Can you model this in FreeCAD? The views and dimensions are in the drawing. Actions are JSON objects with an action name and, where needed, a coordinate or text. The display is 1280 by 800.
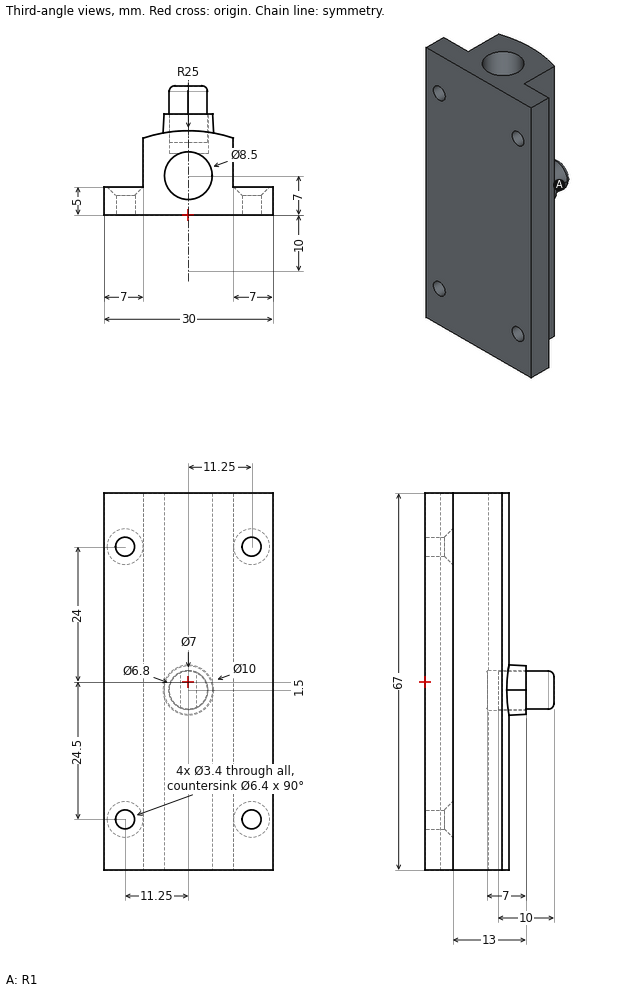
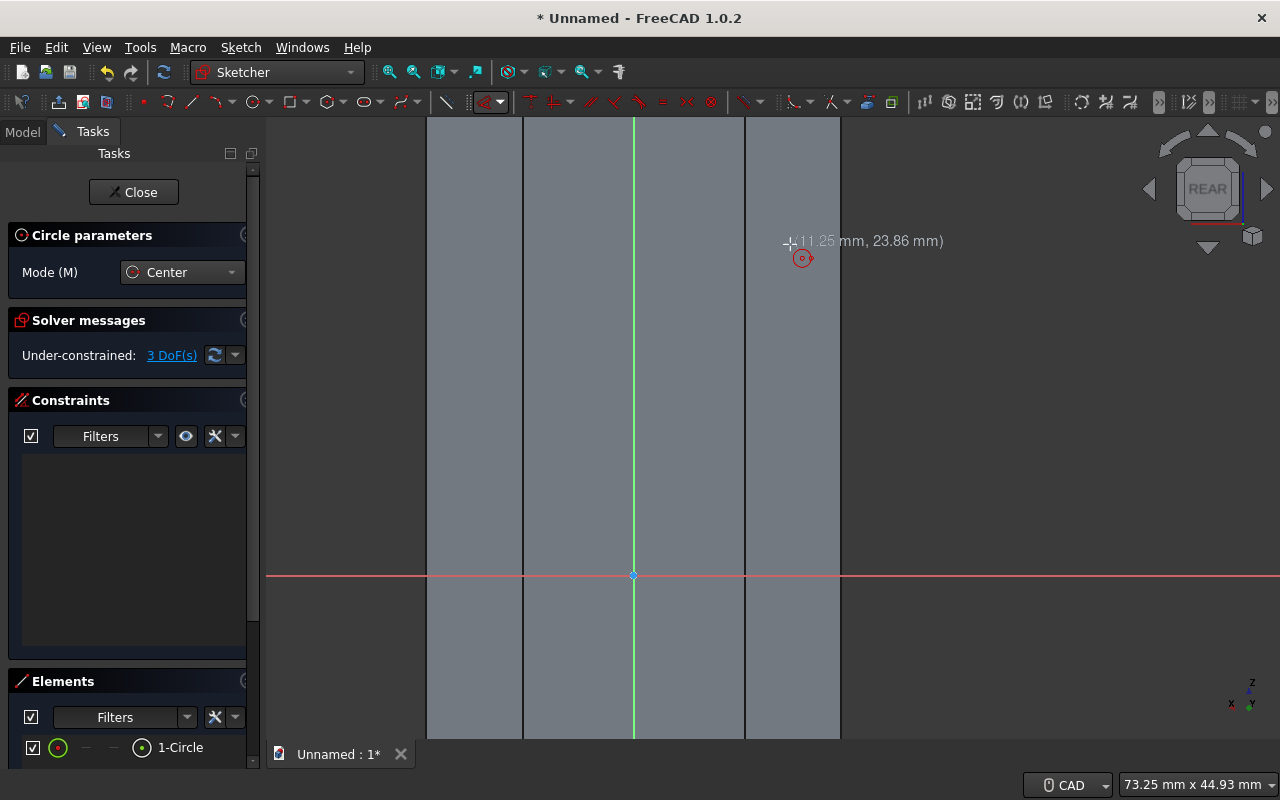
{"action": "left_click", "coordinate": [790, 244]}
{"action": "left_click", "coordinate": [806, 227]}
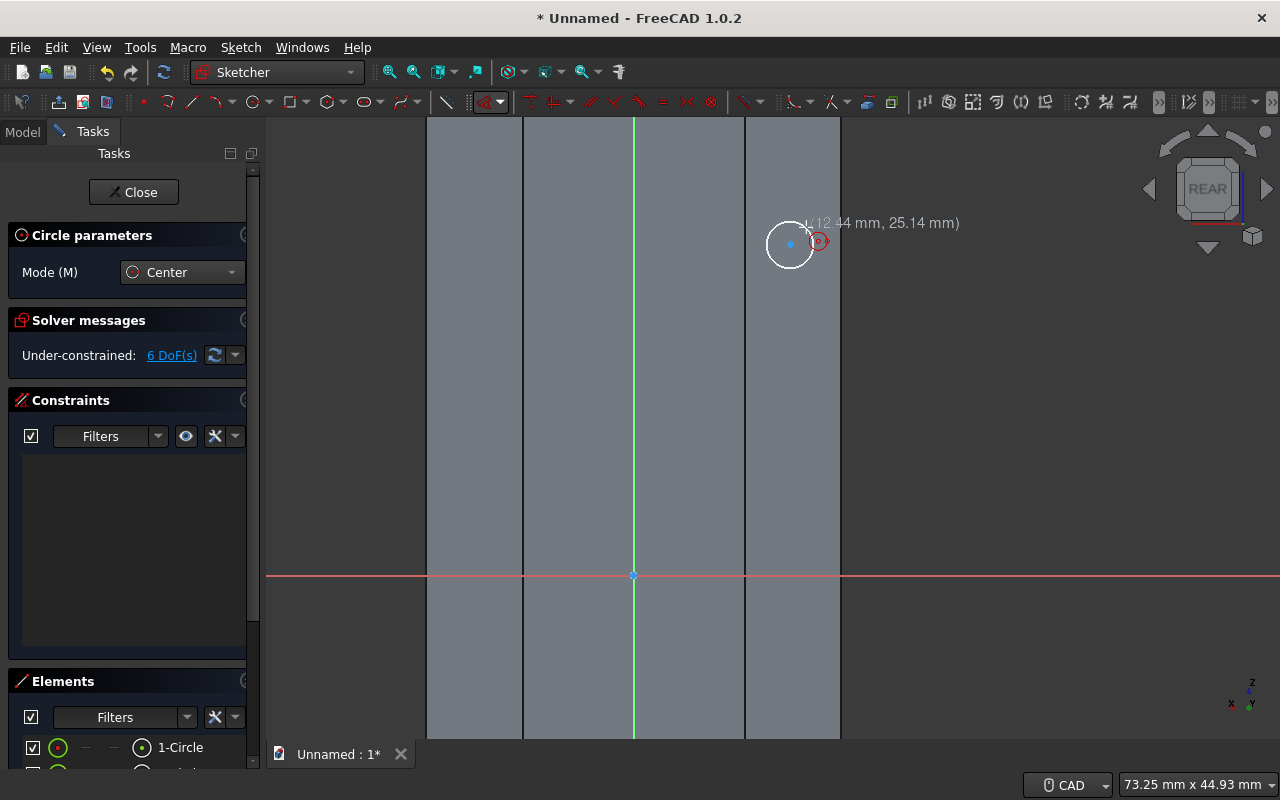
{"action": "left_click", "coordinate": [478, 244]}
{"action": "left_click", "coordinate": [495, 227]}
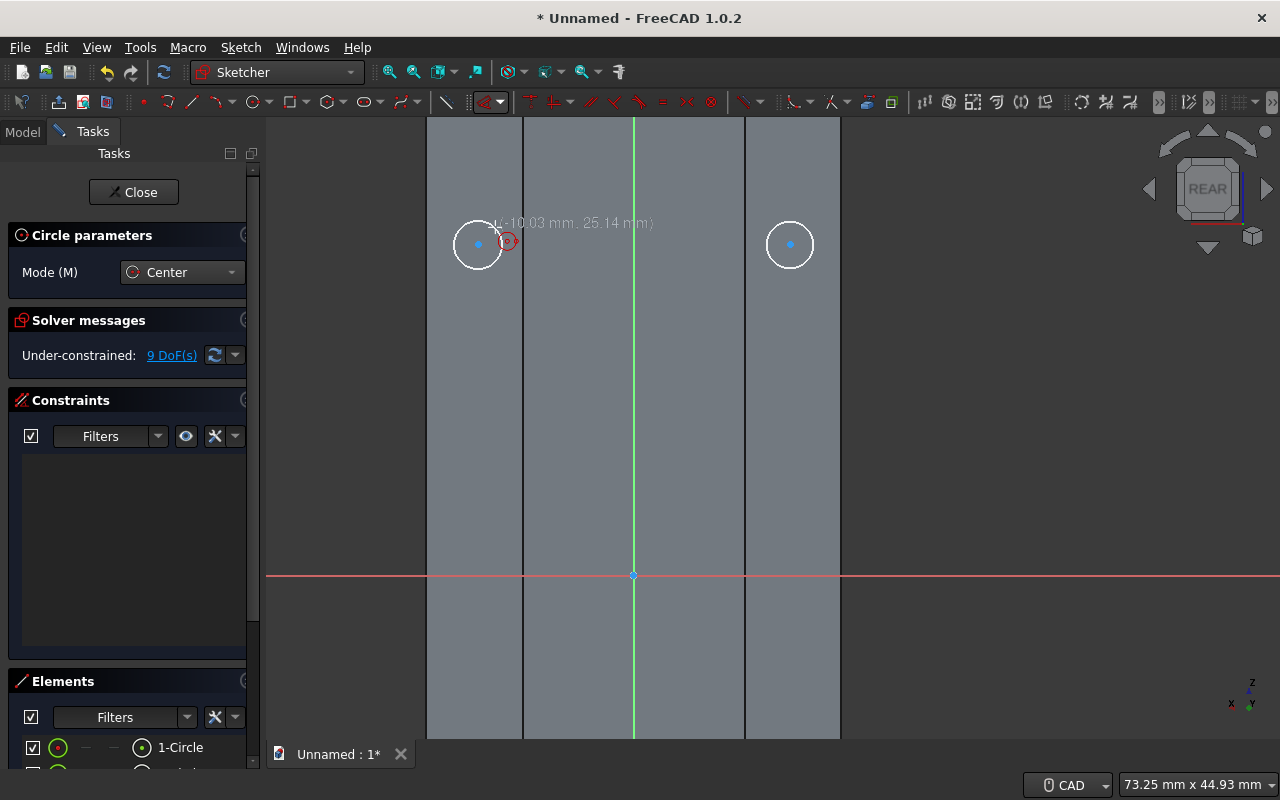
{"action": "scroll", "coordinate": [790, 244], "scroll_direction": "down", "scroll_amount": 3}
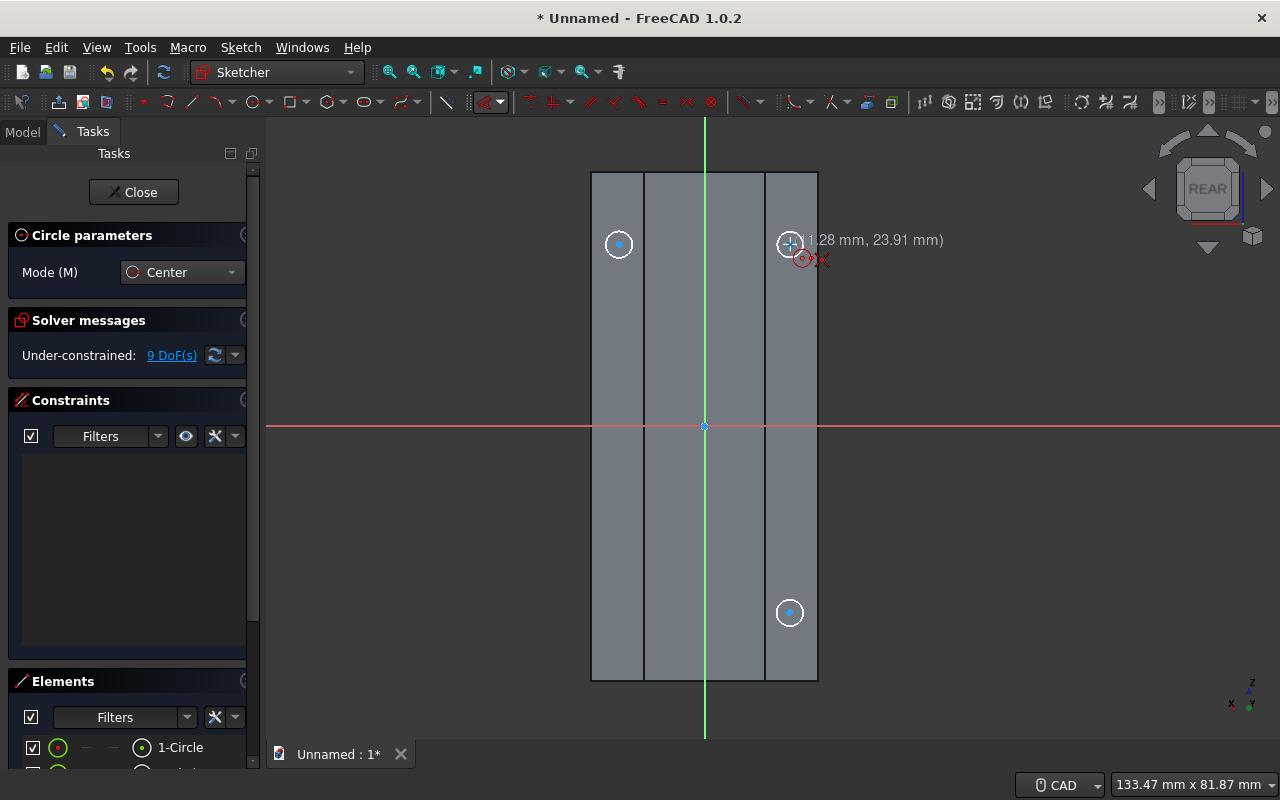
{"action": "scroll", "coordinate": [619, 612], "scroll_direction": "up", "scroll_amount": 3}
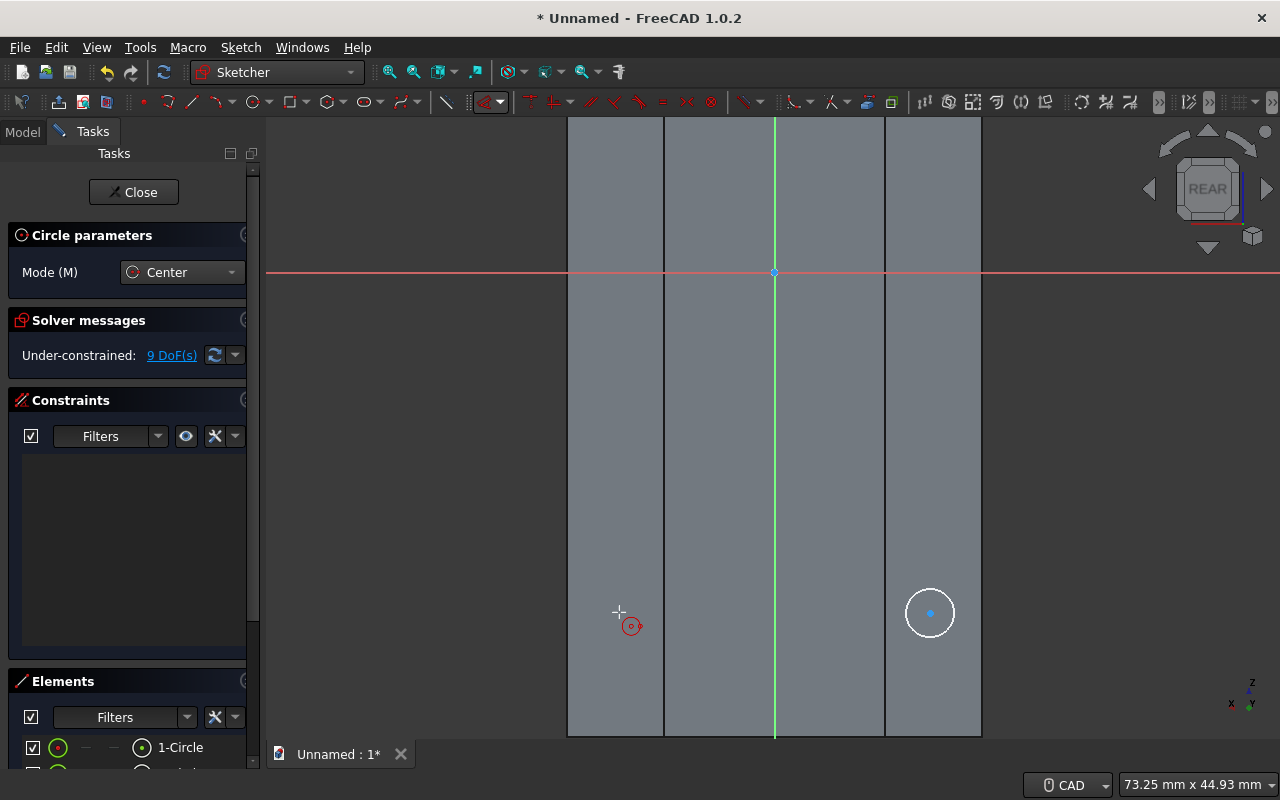
{"action": "left_click", "coordinate": [619, 612]}
{"action": "left_click", "coordinate": [635, 595]}
{"action": "key", "text": "Escape"}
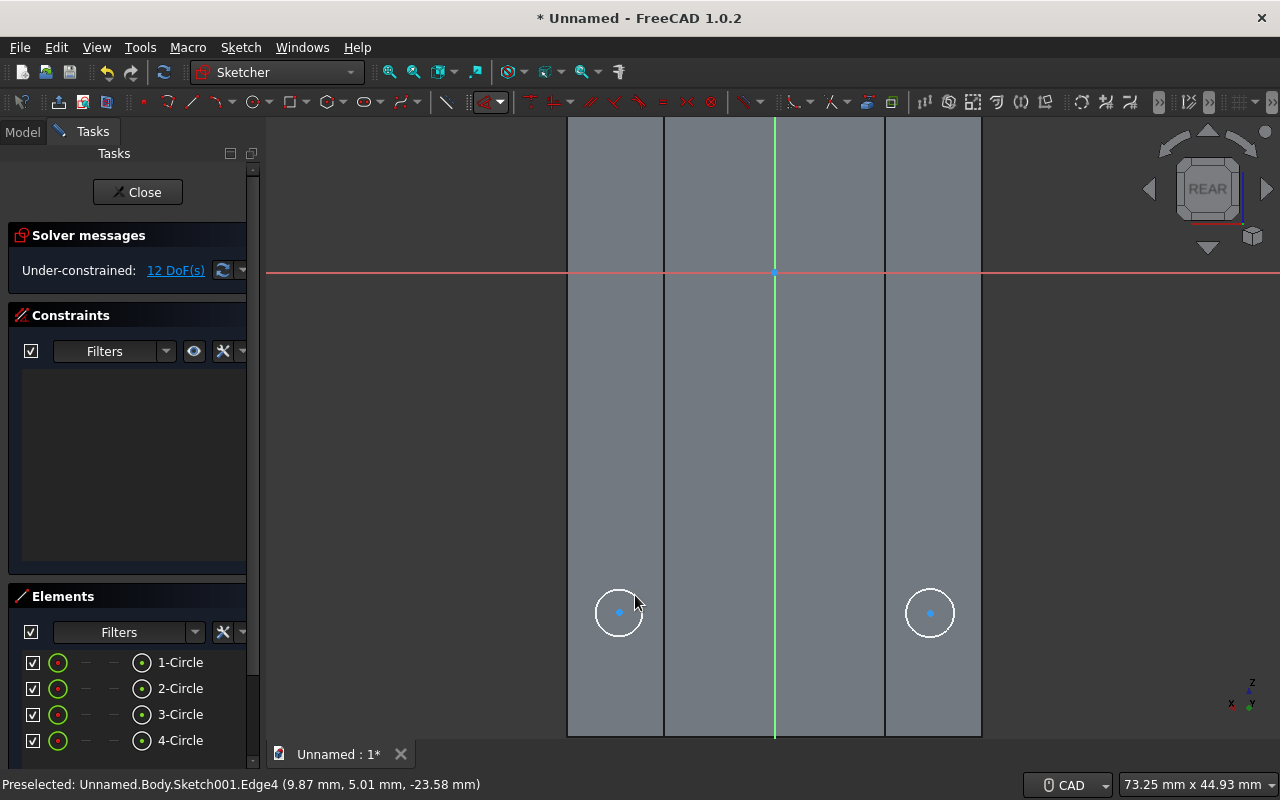
{"action": "left_click", "coordinate": [947, 596]}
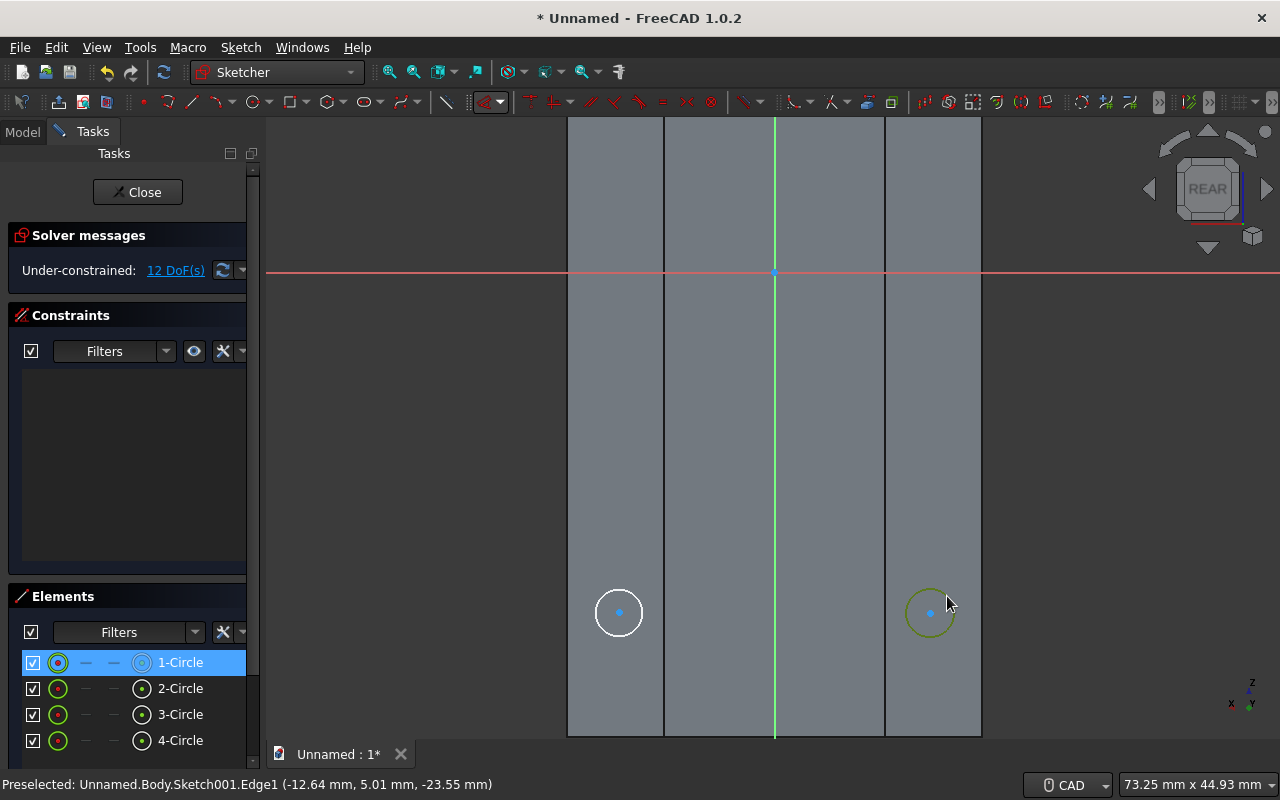
{"action": "scroll", "coordinate": [619, 612], "scroll_direction": "down", "scroll_amount": 3}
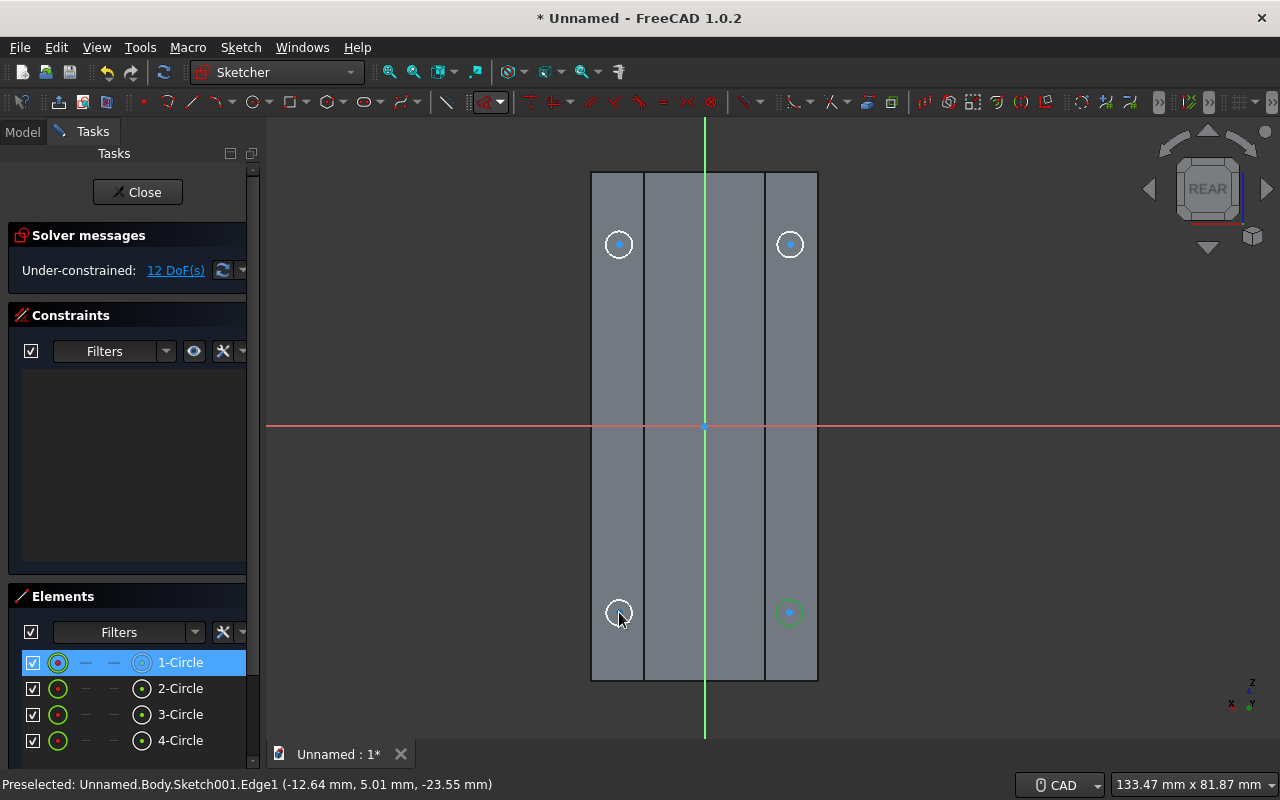
{"action": "left_click", "coordinate": [799, 236]}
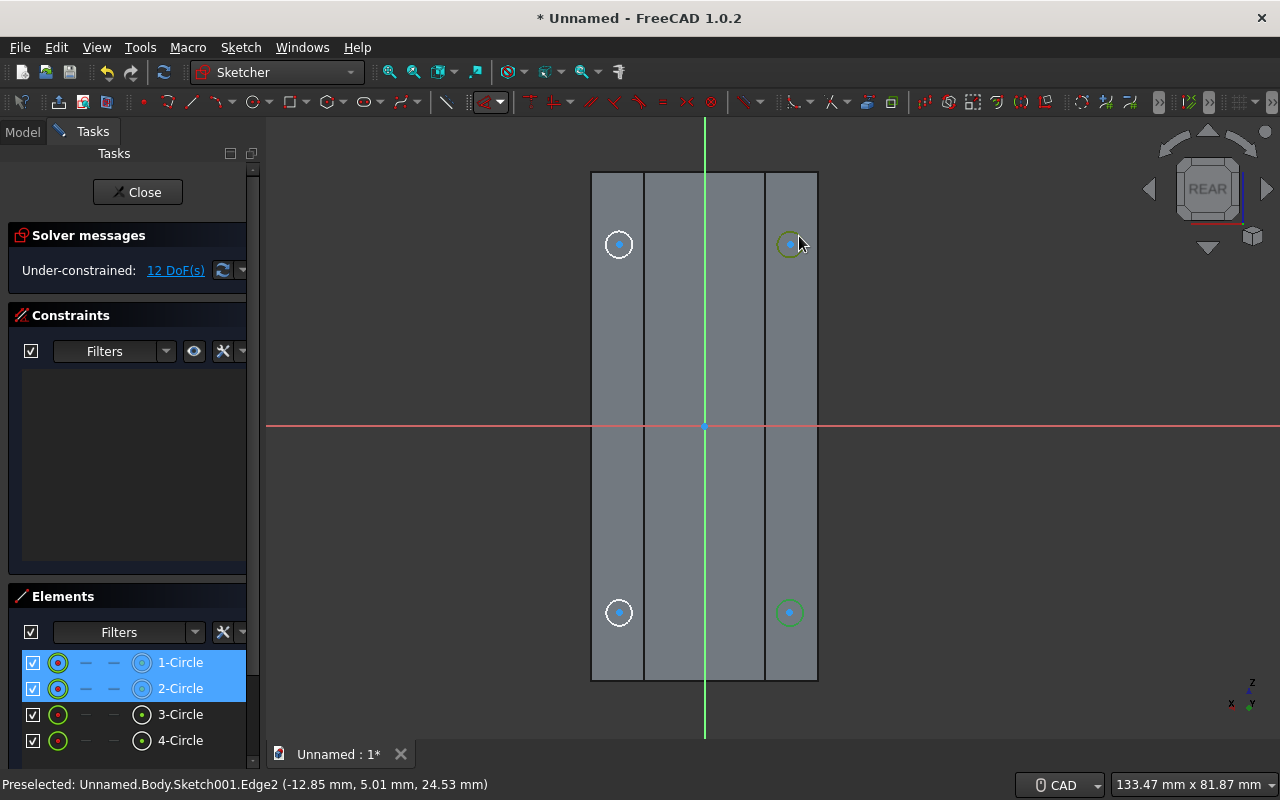
{"action": "left_click", "coordinate": [628, 235]}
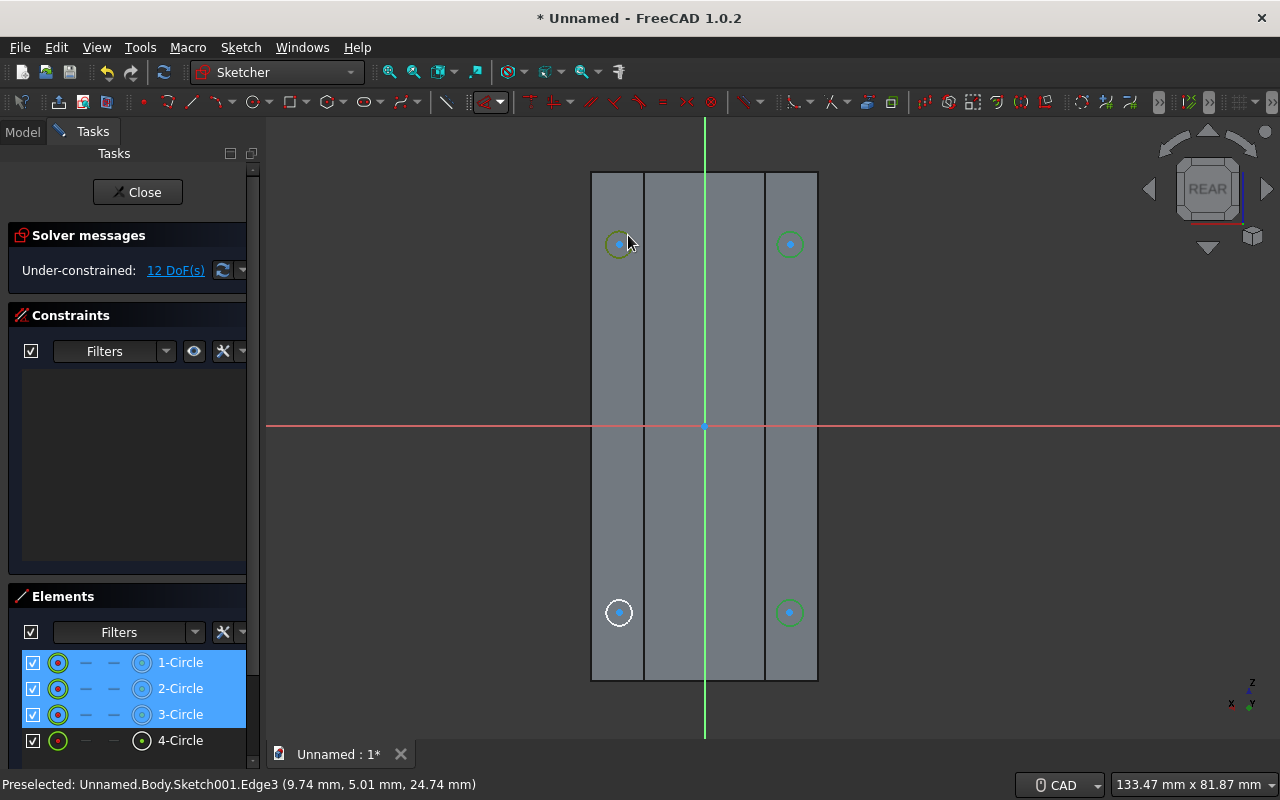
{"action": "left_click", "coordinate": [628, 604]}